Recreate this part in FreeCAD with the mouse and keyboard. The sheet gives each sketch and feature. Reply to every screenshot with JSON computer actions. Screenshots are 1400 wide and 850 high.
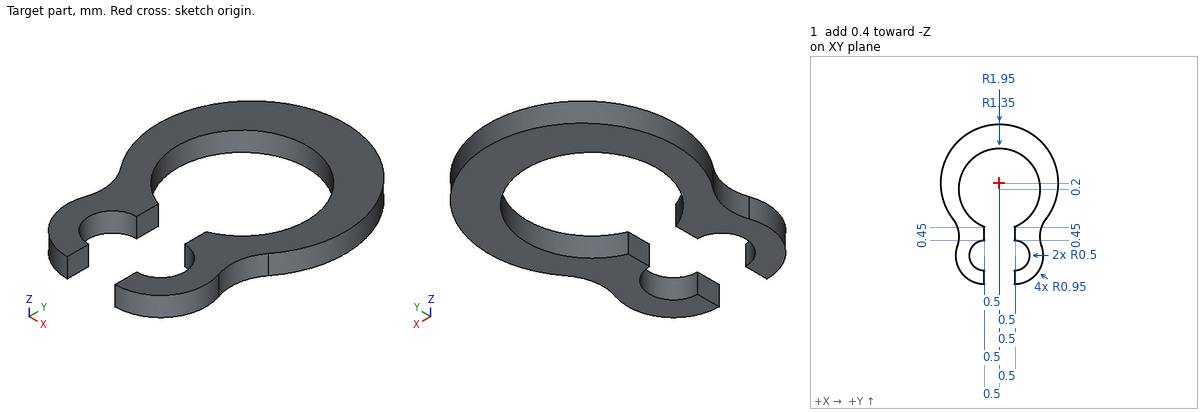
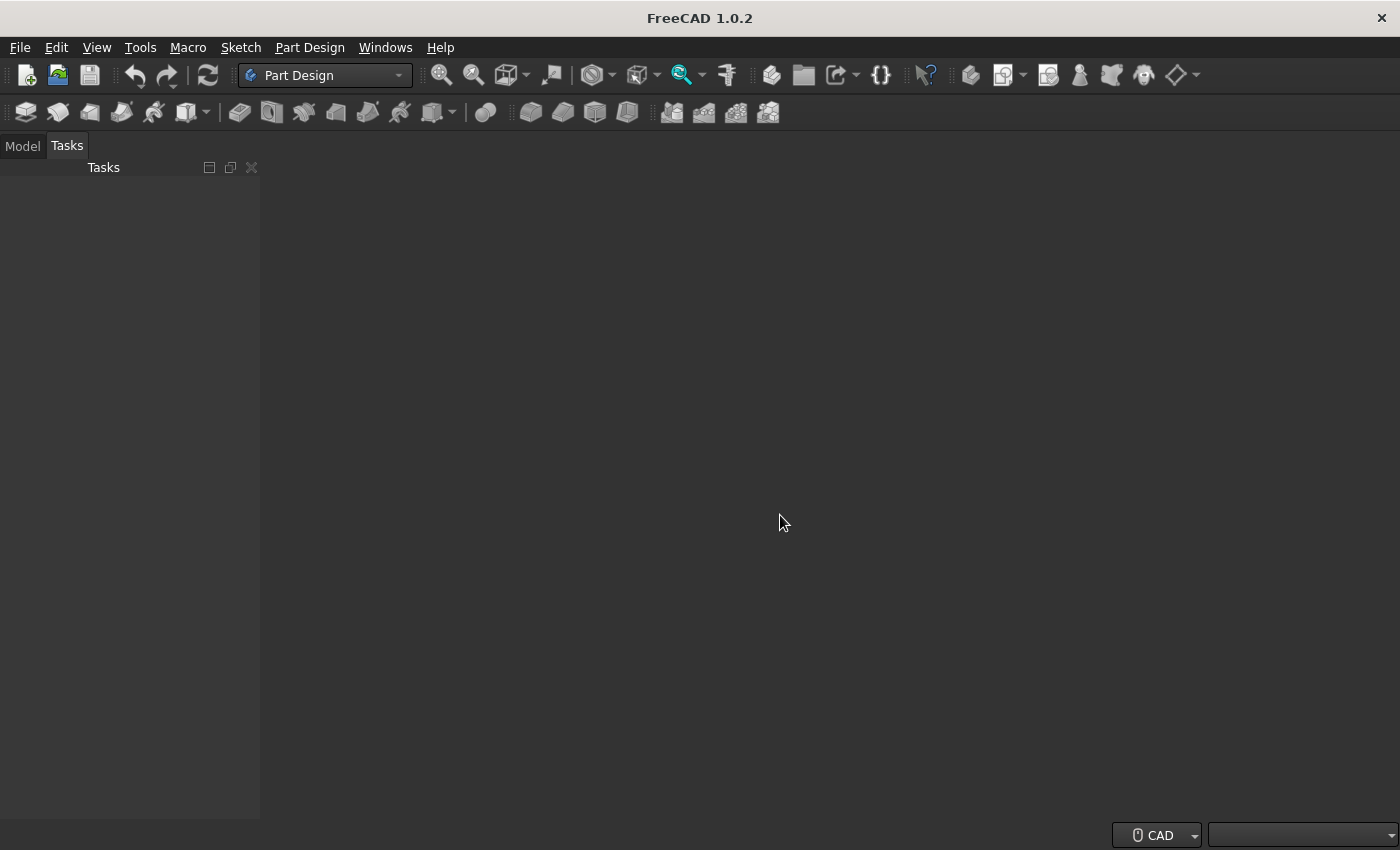
{"action": "key", "text": "ctrl+n"}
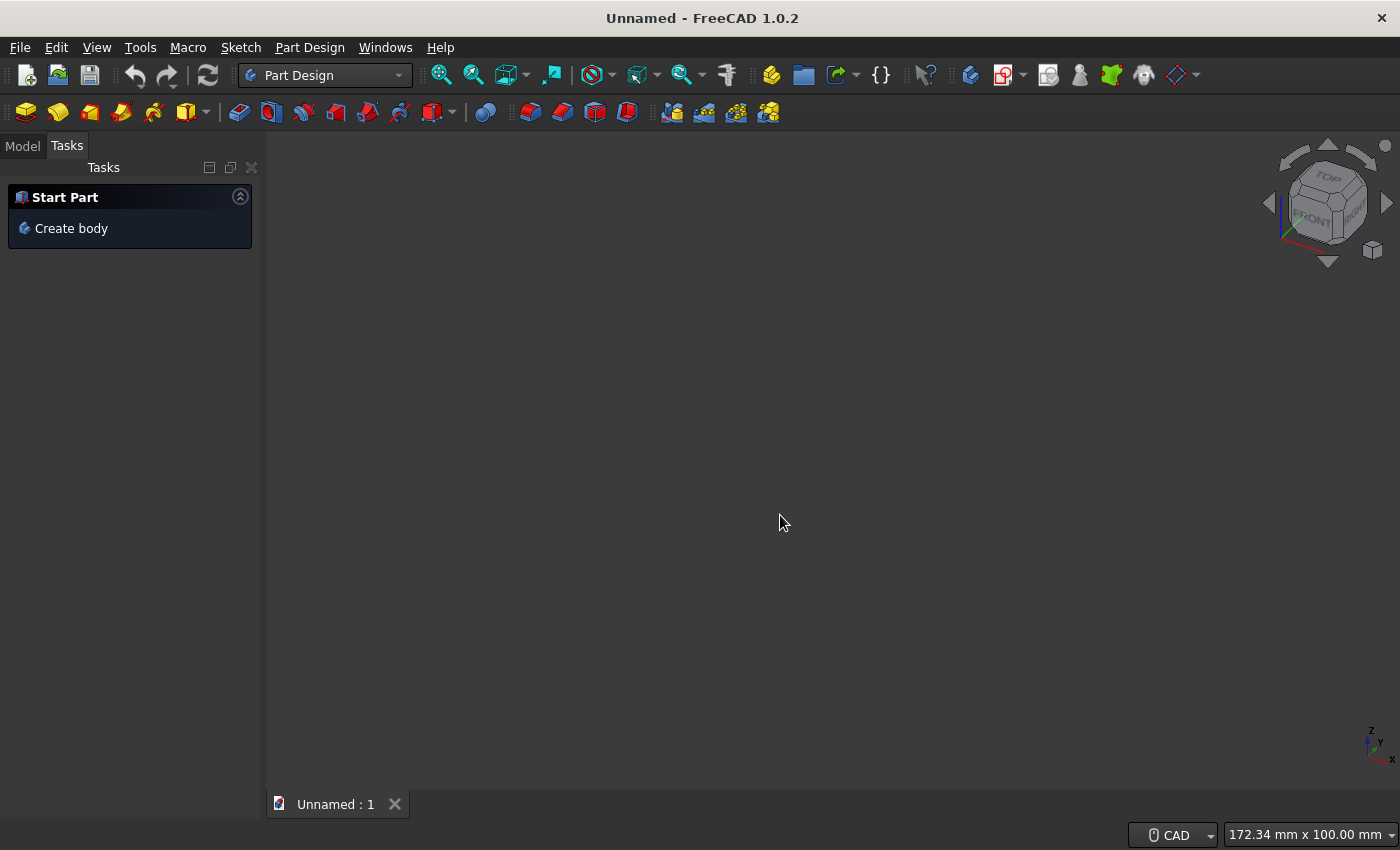
{"action": "left_click", "coordinate": [1004, 76]}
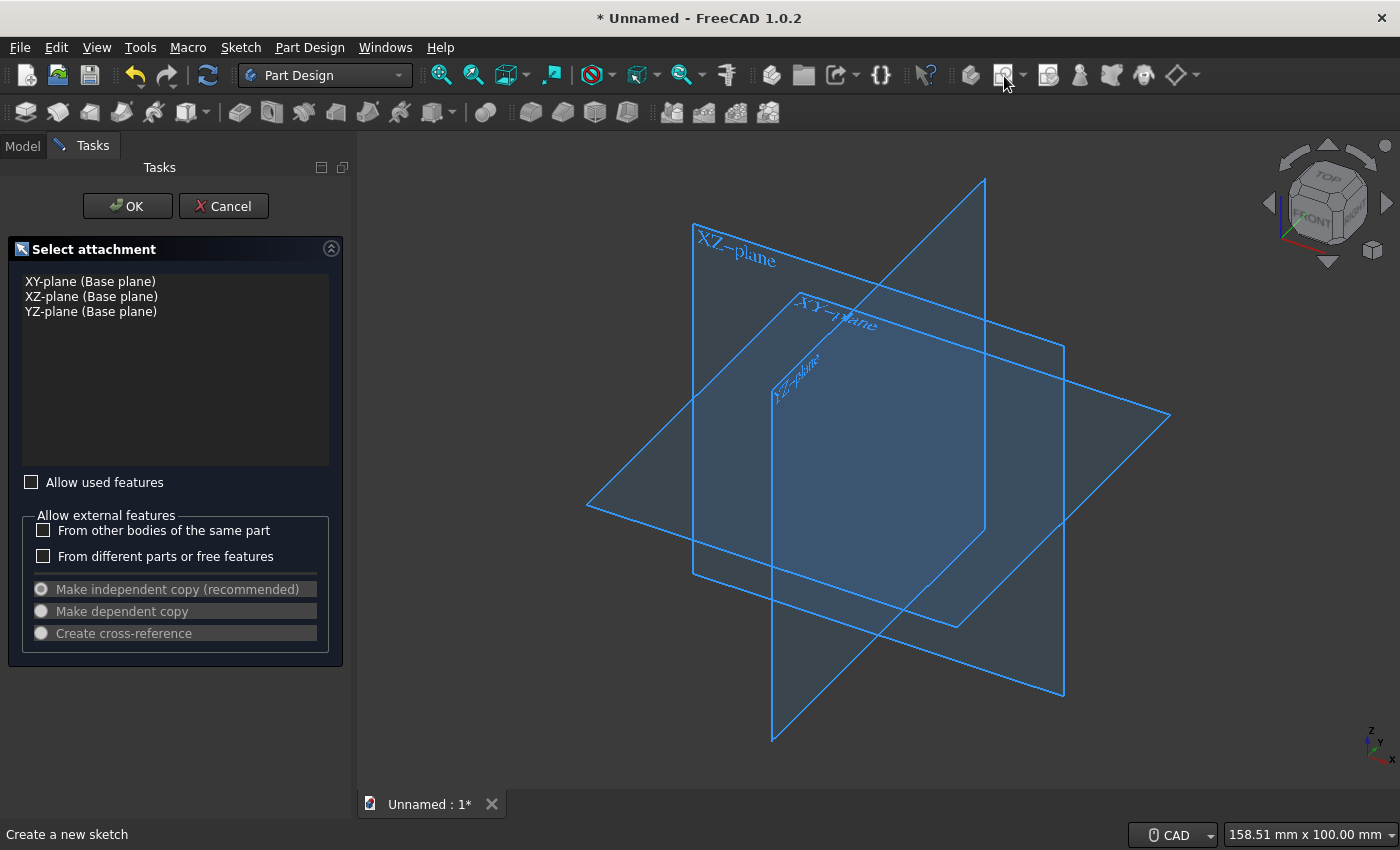
{"action": "left_click", "coordinate": [82, 282]}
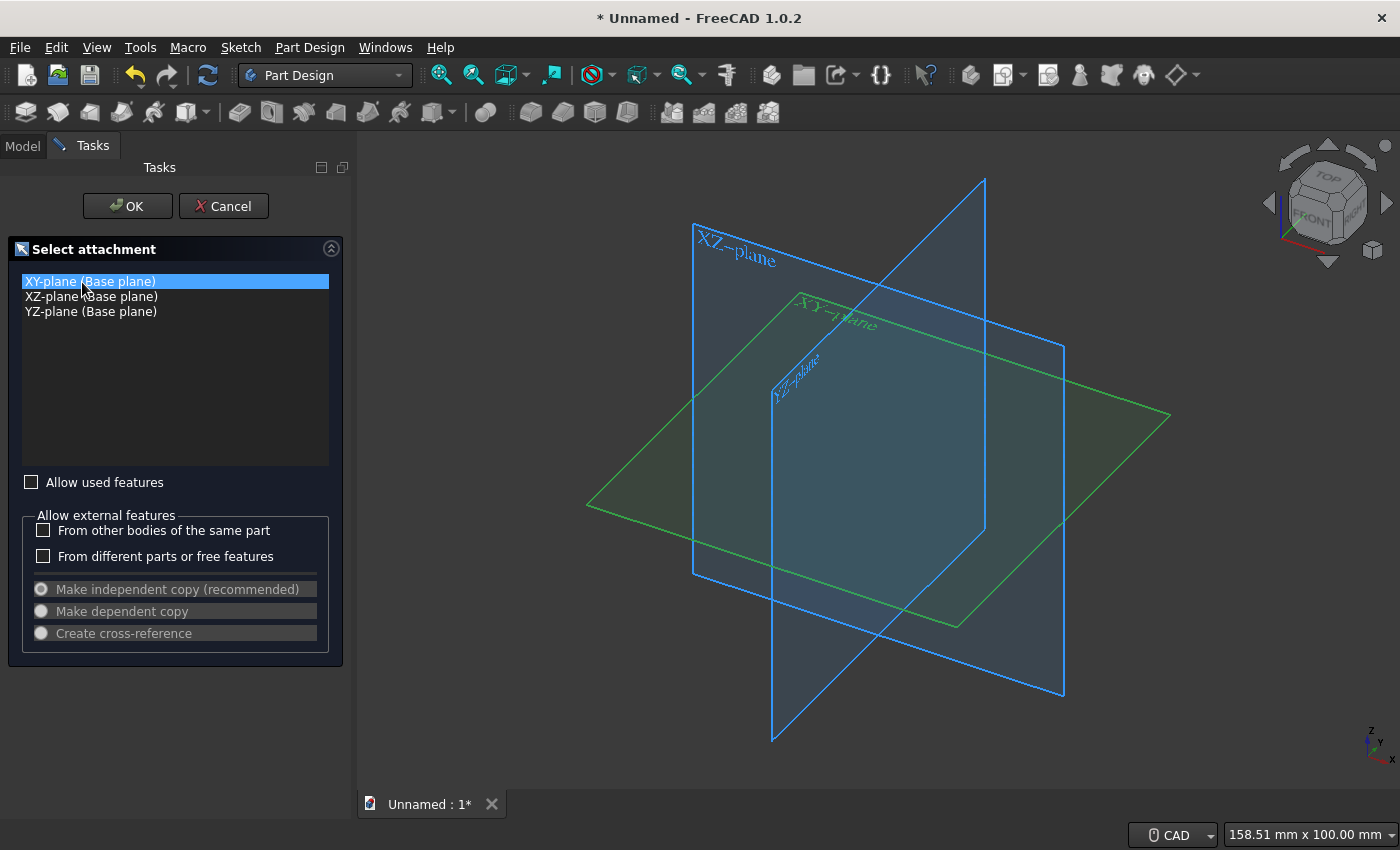
{"action": "left_click", "coordinate": [128, 206]}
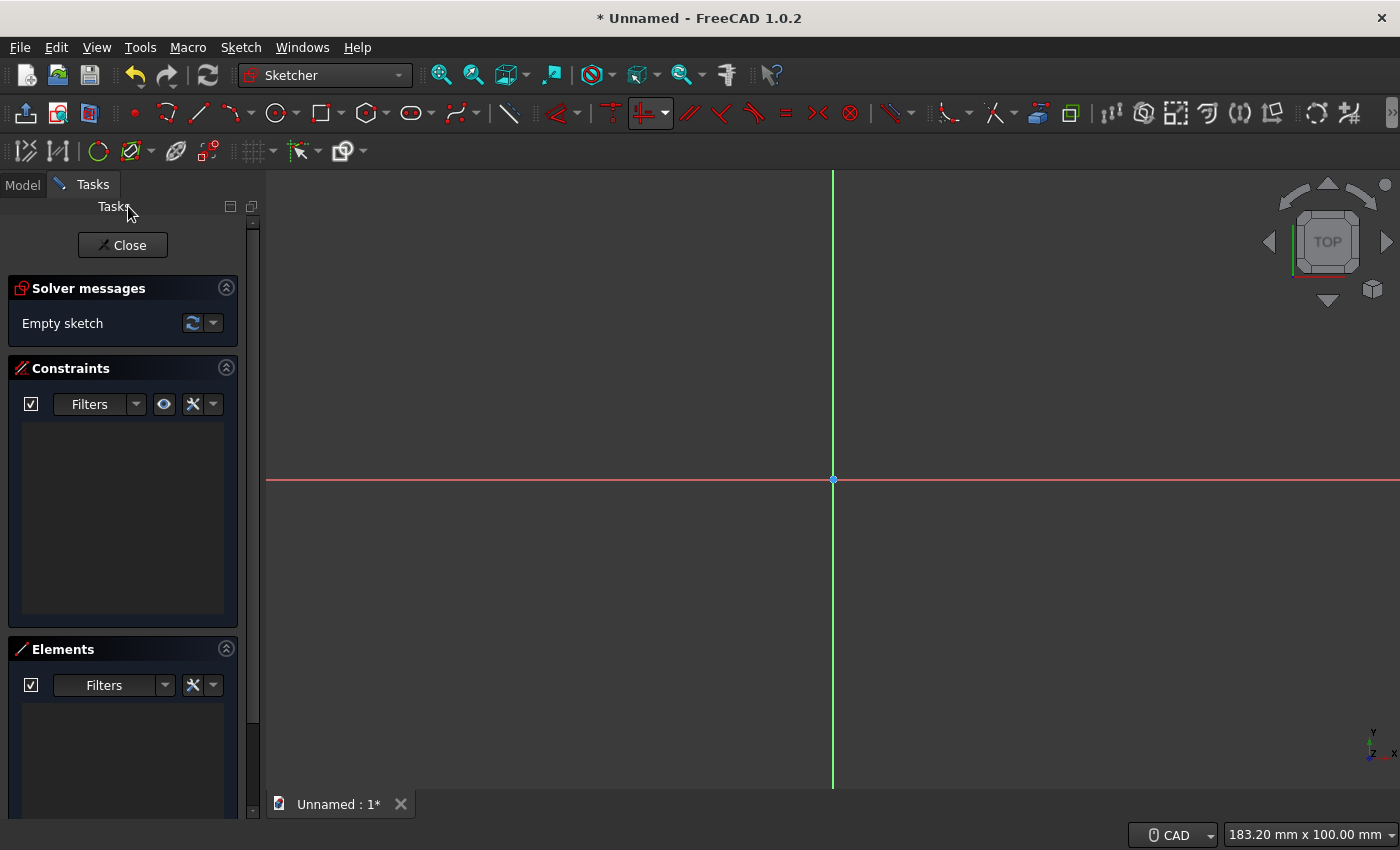
{"action": "scroll", "coordinate": [840, 484], "scroll_direction": "up", "scroll_amount": 12}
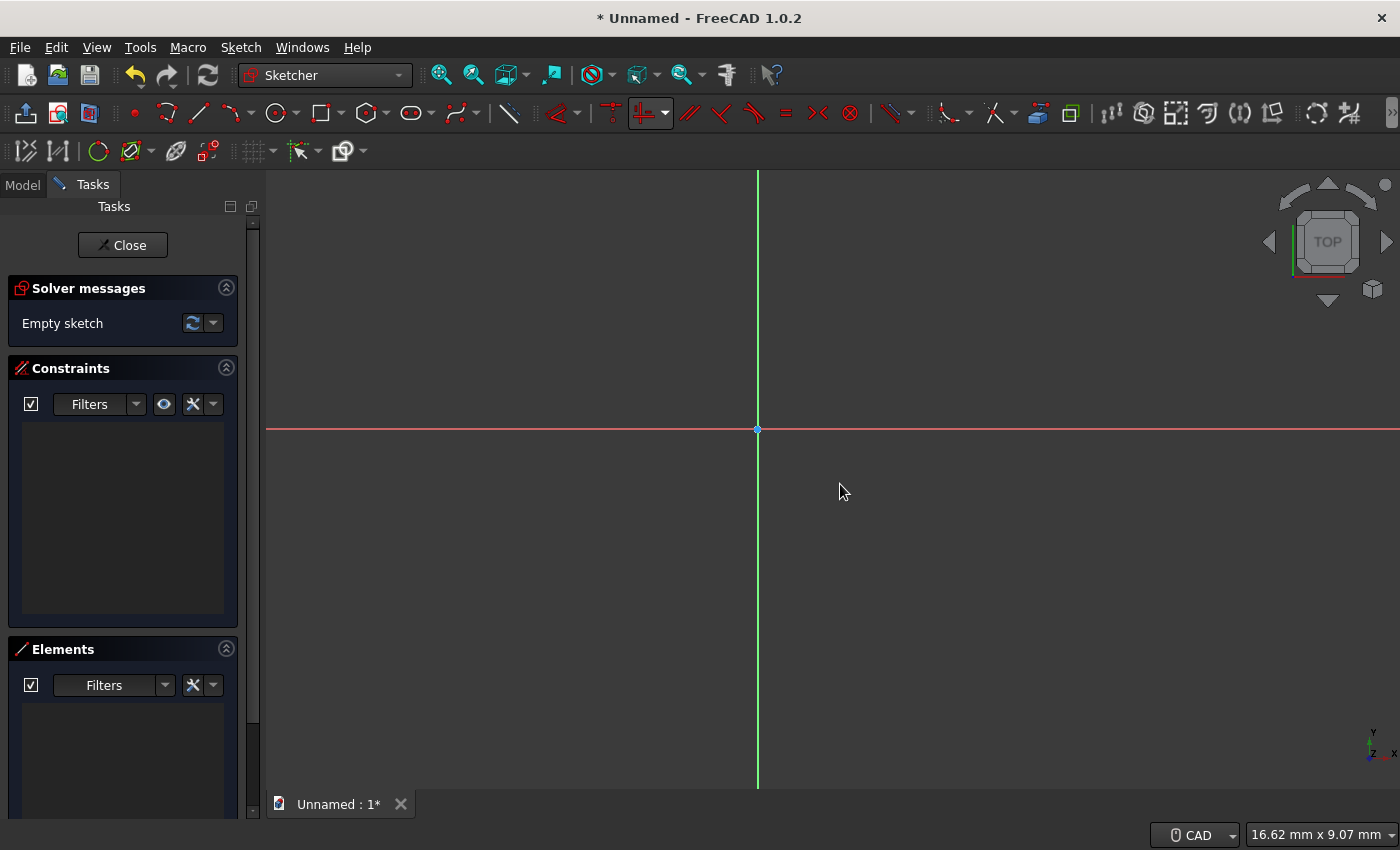
{"action": "left_click", "coordinate": [200, 114]}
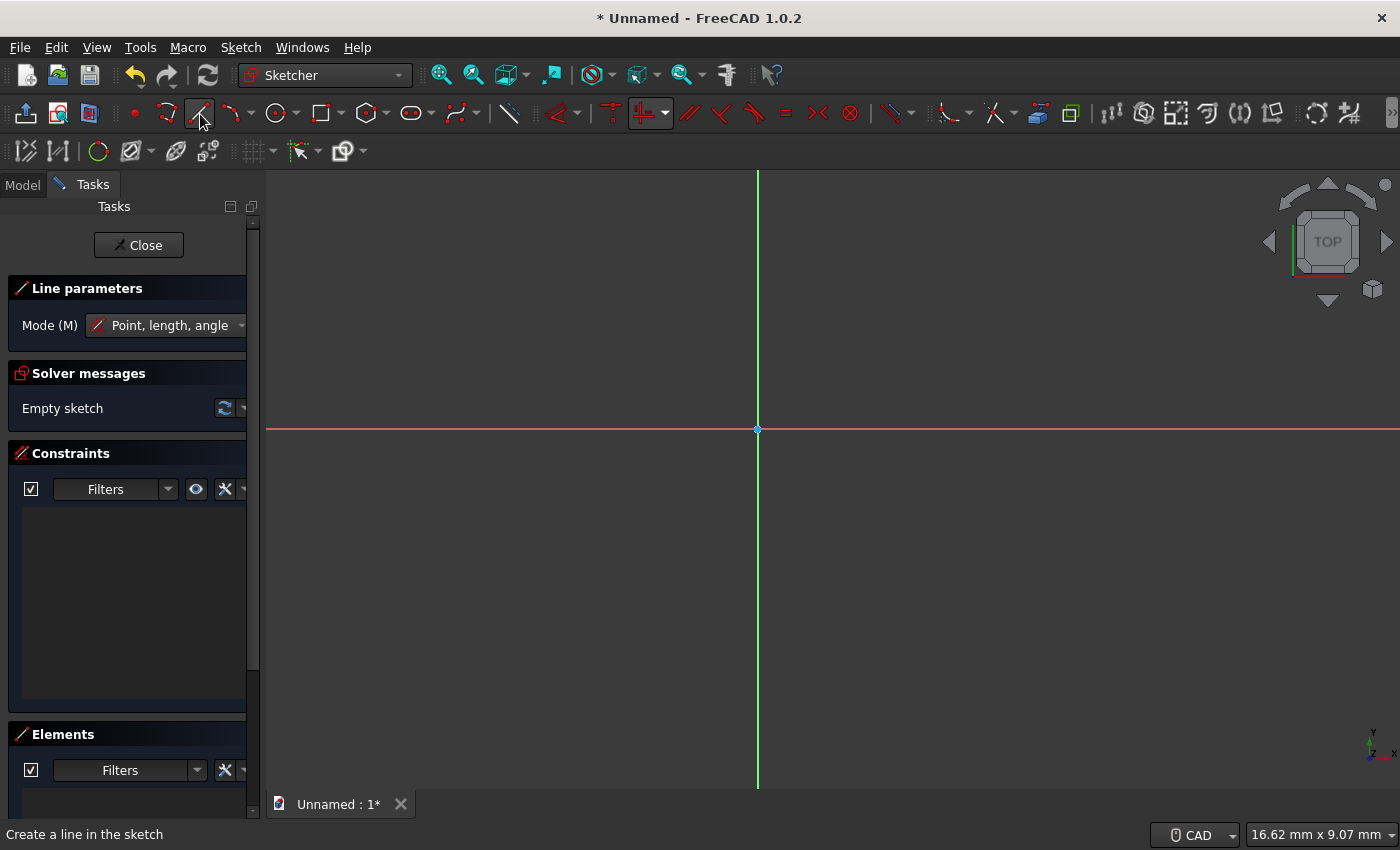
{"action": "left_click", "coordinate": [724, 559]}
{"action": "left_click", "coordinate": [724, 529]}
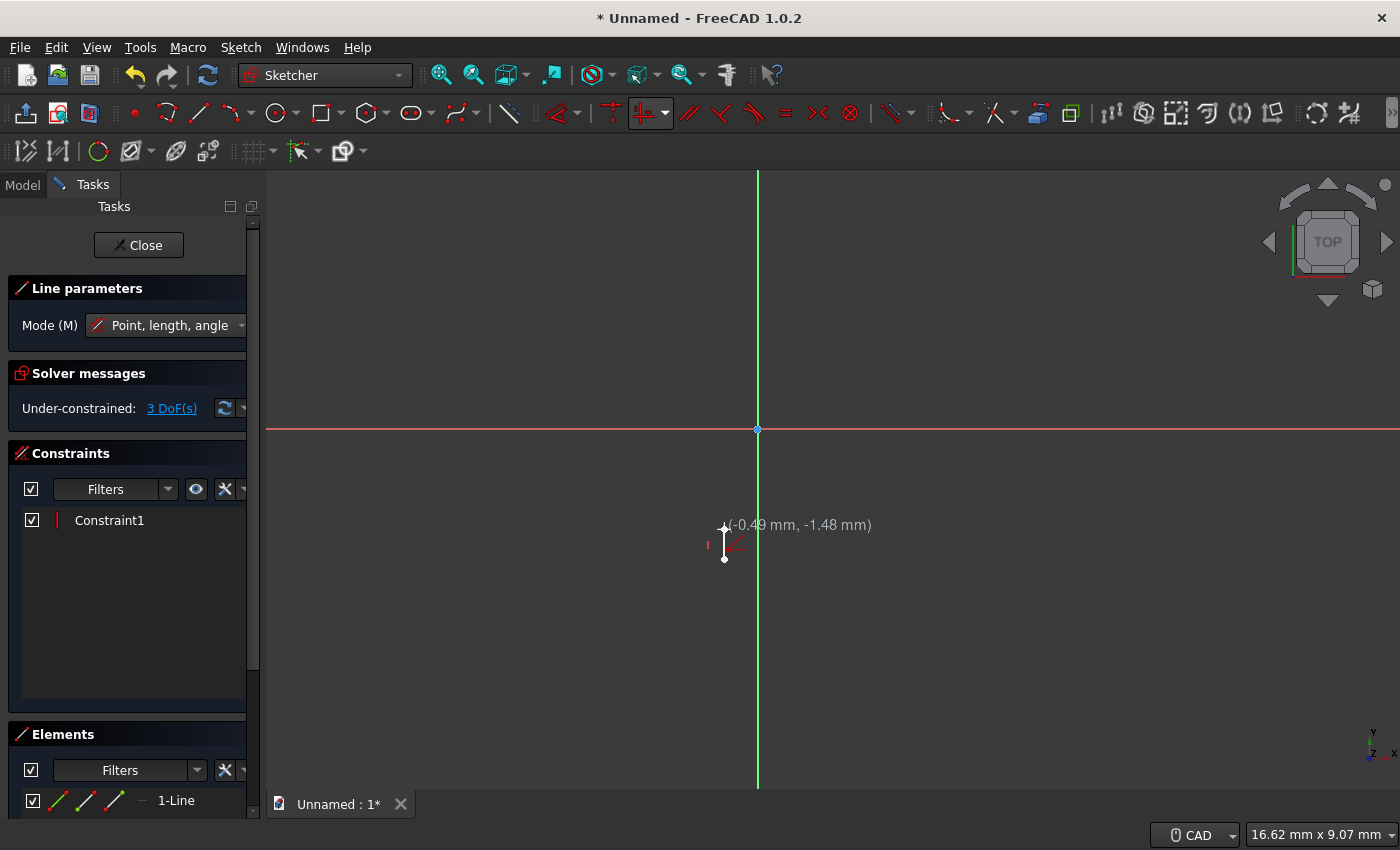
{"action": "left_click", "coordinate": [792, 529]}
{"action": "left_click", "coordinate": [792, 559]}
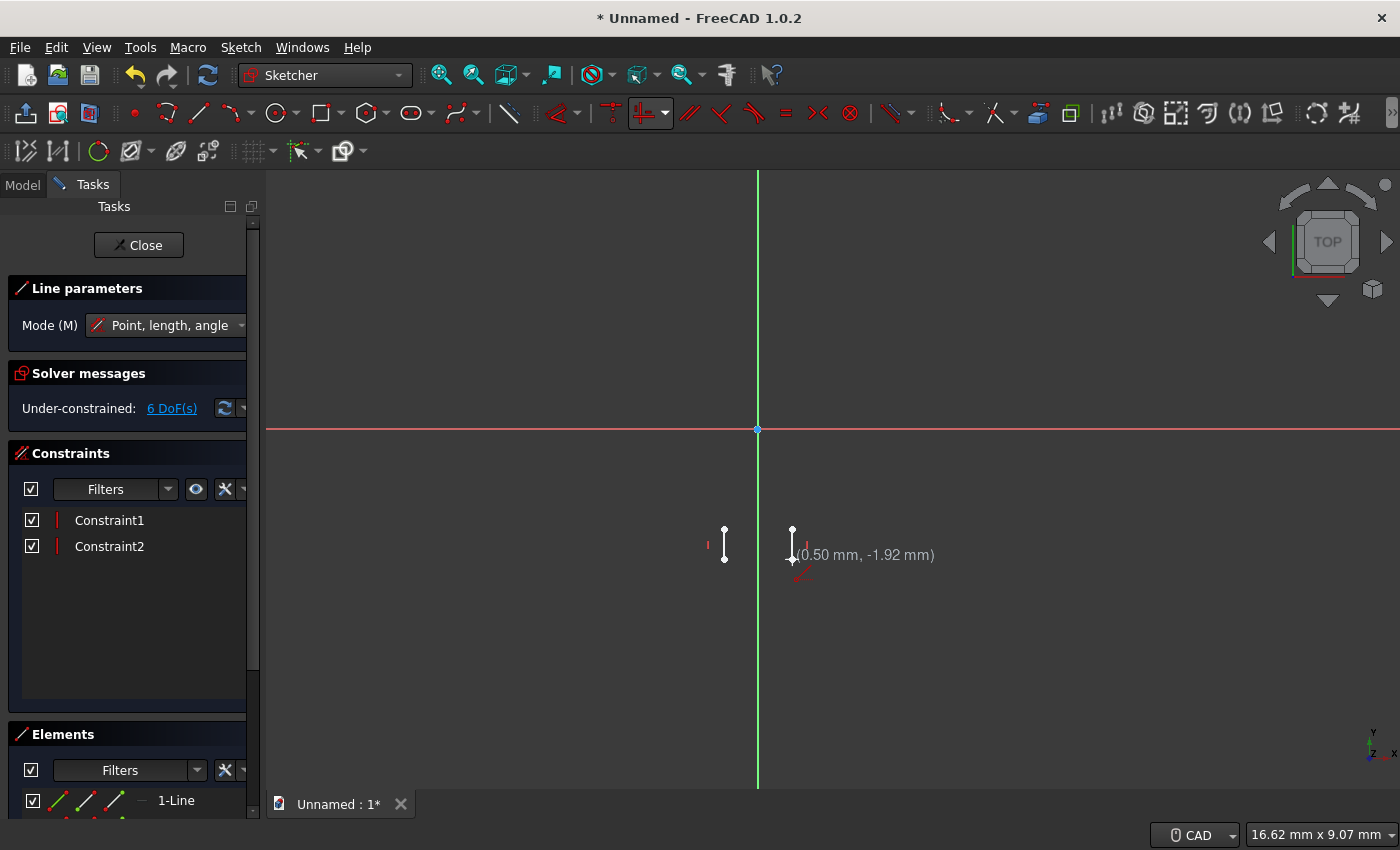
{"action": "left_click", "coordinate": [792, 627]}
{"action": "left_click", "coordinate": [792, 658]}